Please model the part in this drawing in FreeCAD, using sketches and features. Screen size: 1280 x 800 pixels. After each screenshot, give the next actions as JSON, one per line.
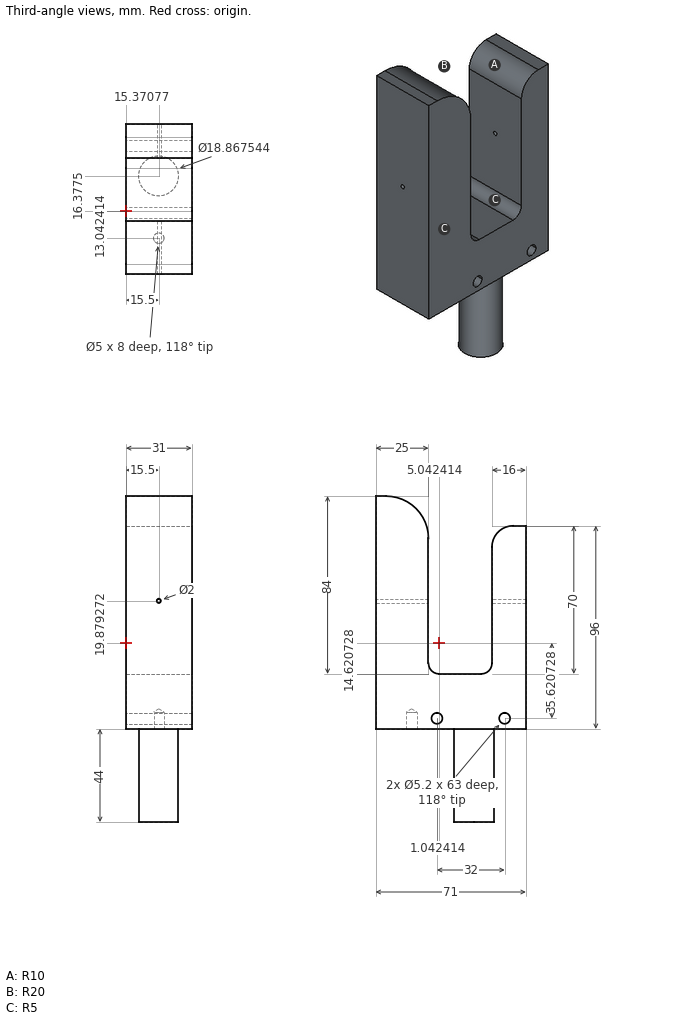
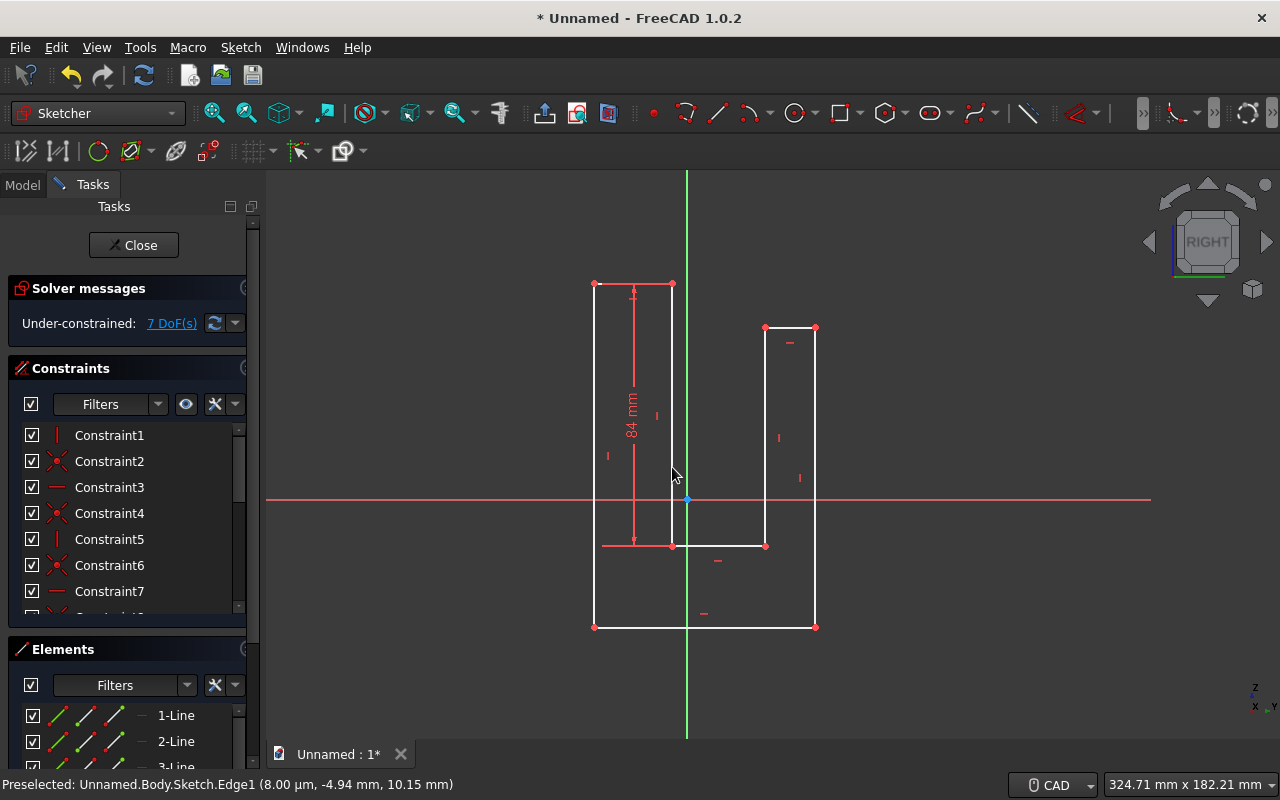
{"action": "left_click", "coordinate": [649, 284]}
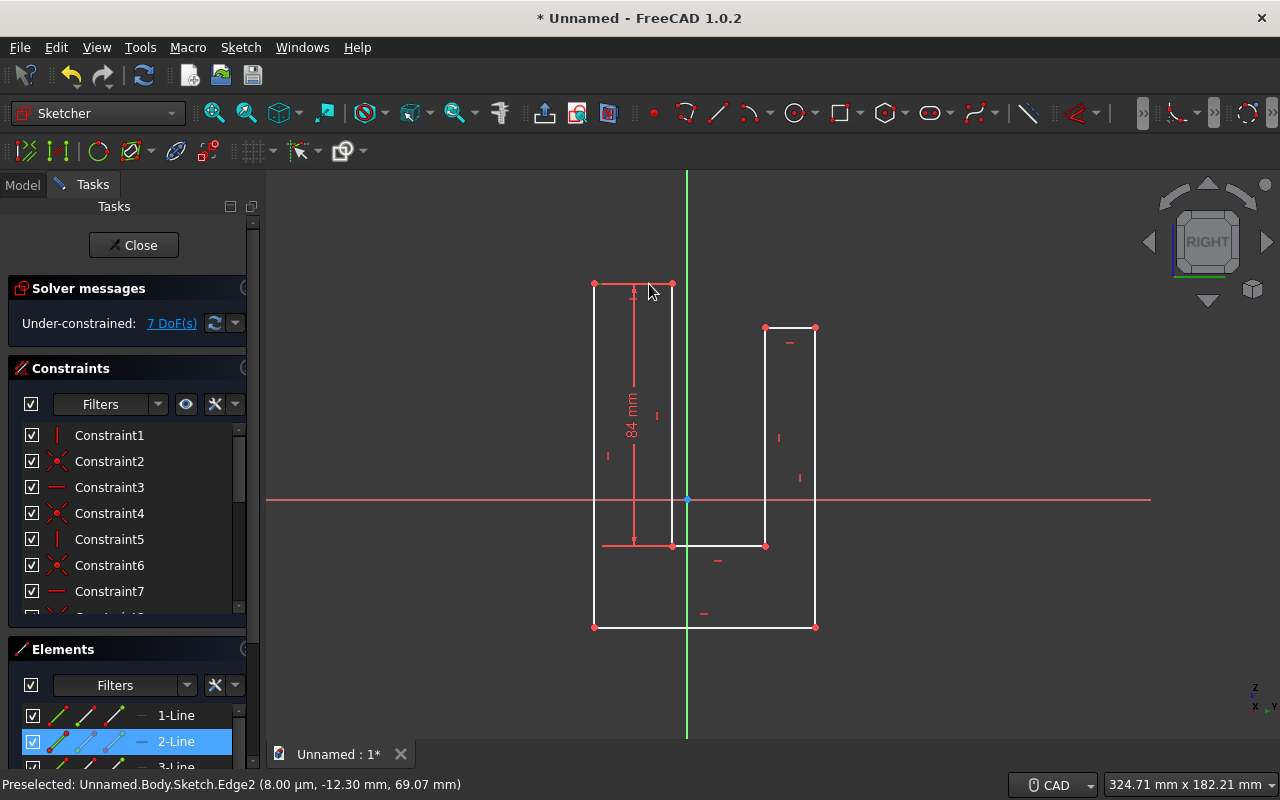
{"action": "left_click", "coordinate": [1098, 114]}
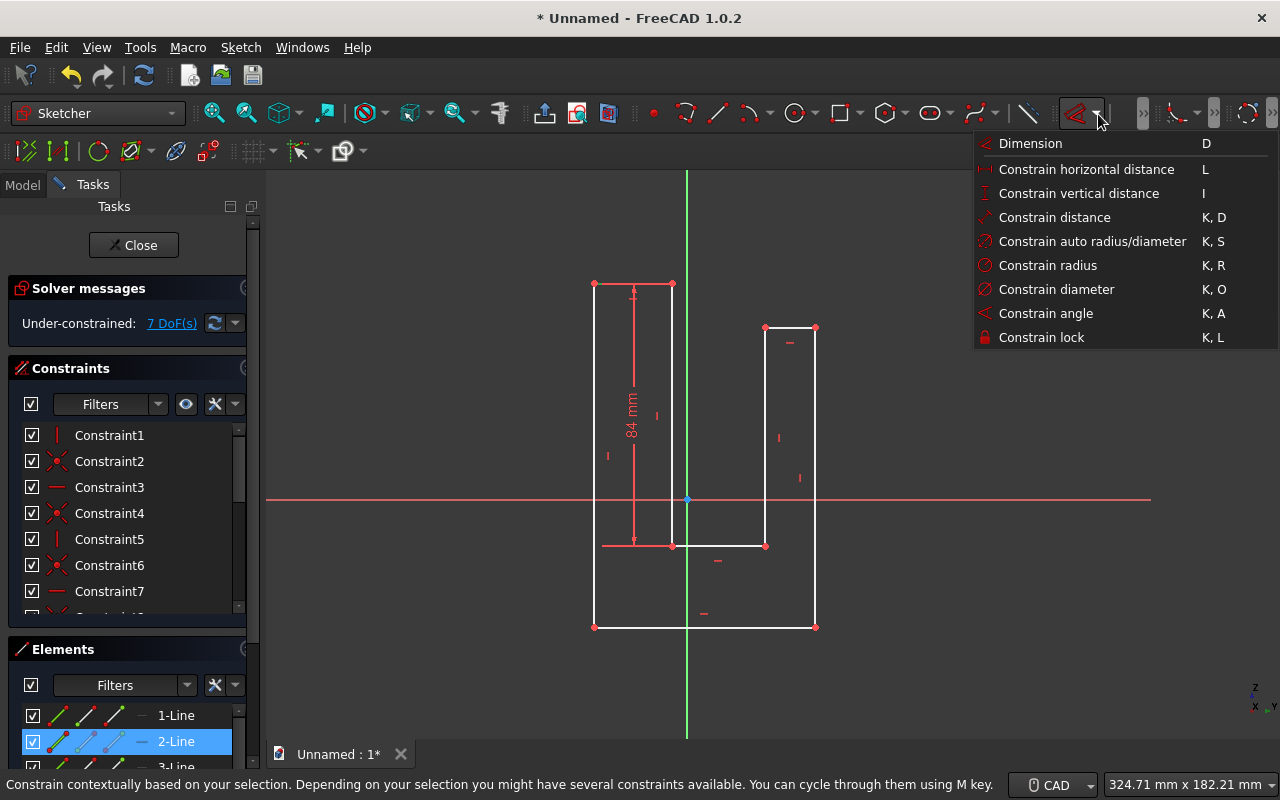
{"action": "left_click", "coordinate": [1126, 169]}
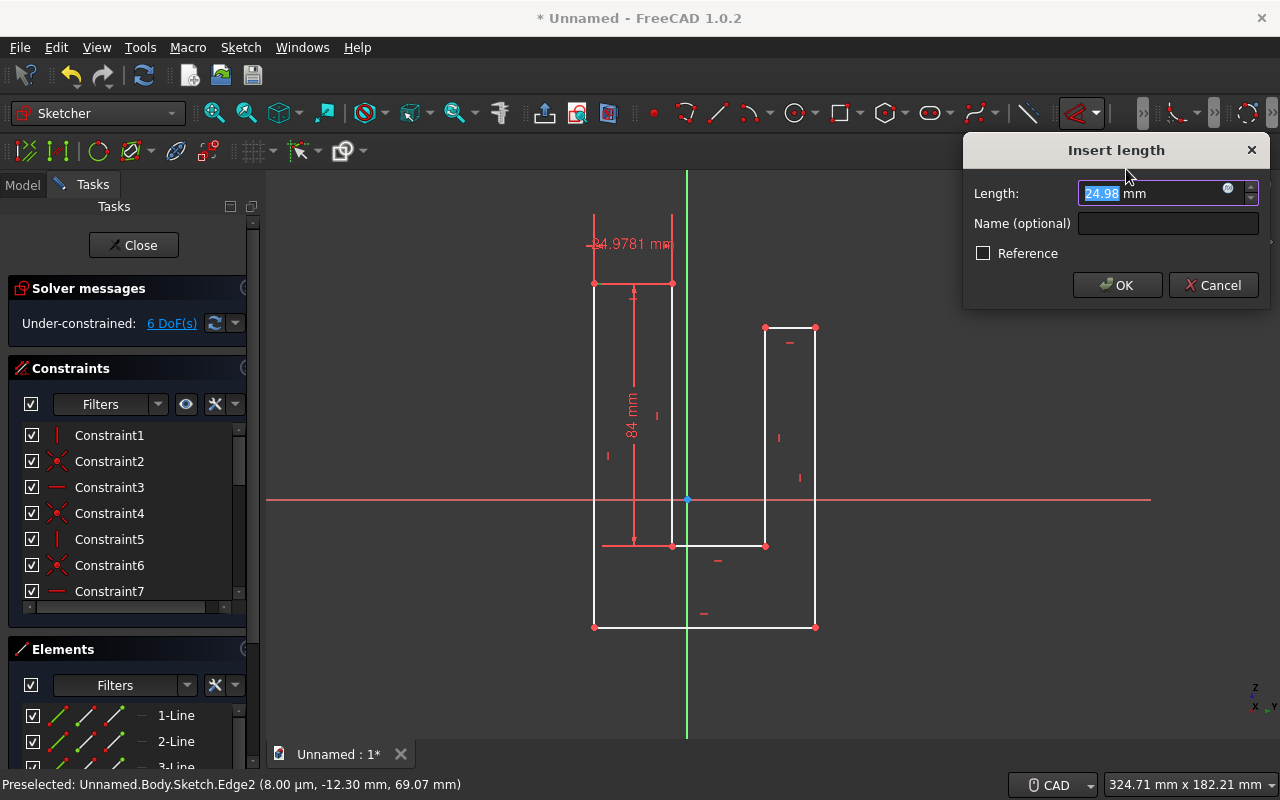
{"action": "type", "text": "25"}
{"action": "key", "text": "Return"}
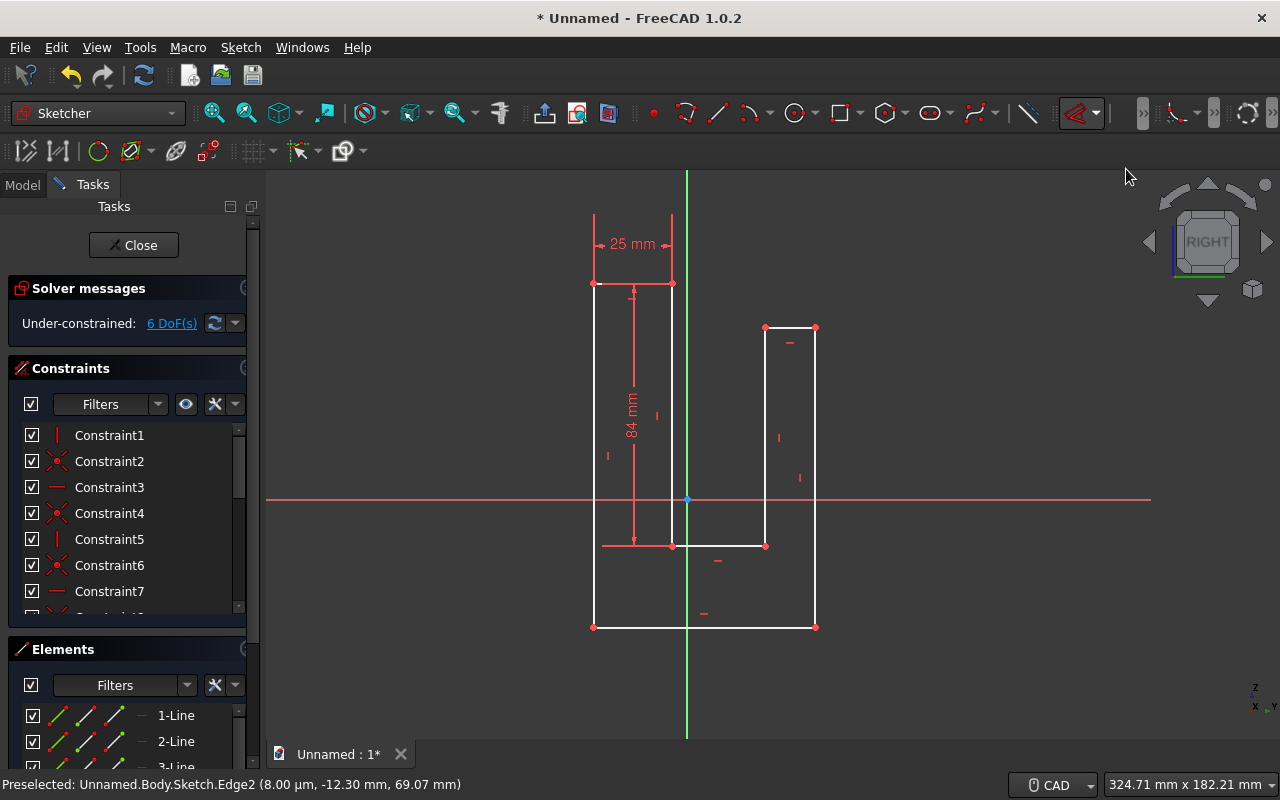
{"action": "left_click", "coordinate": [660, 628]}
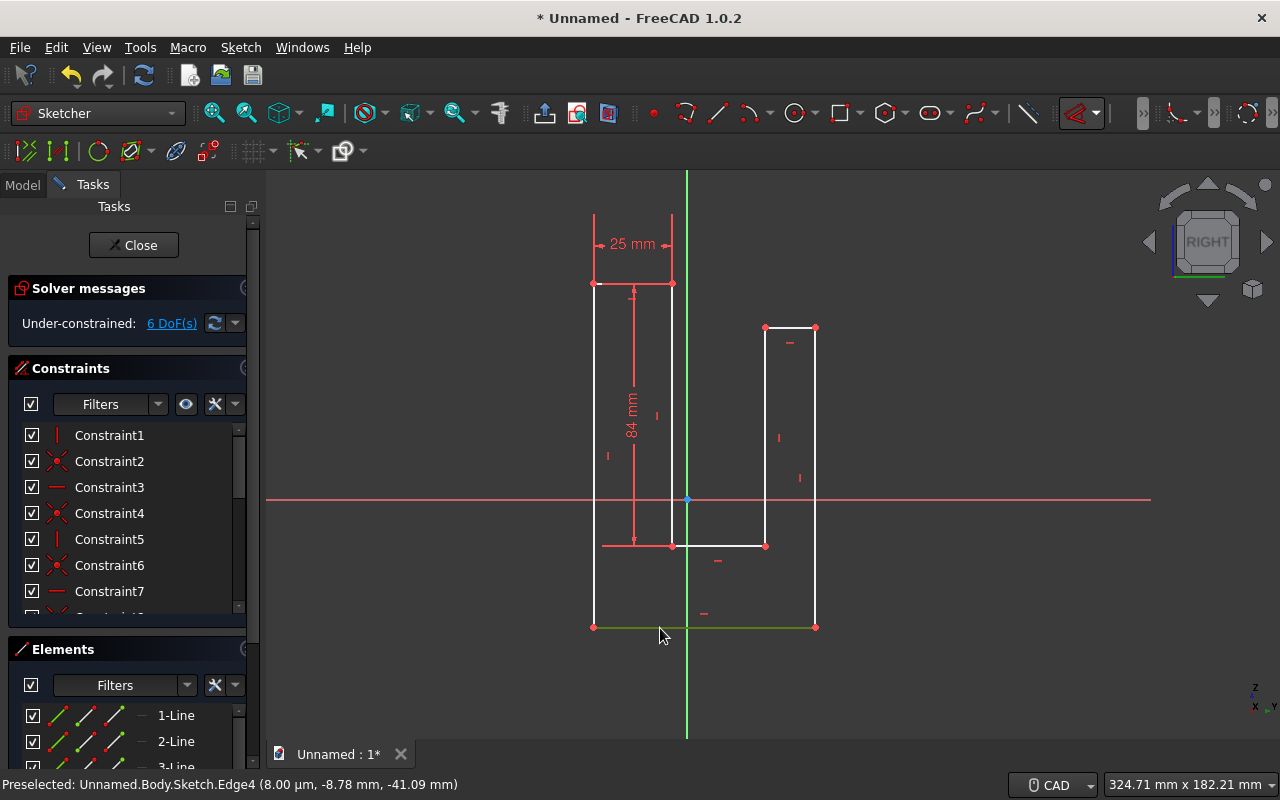
{"action": "key", "text": "l"}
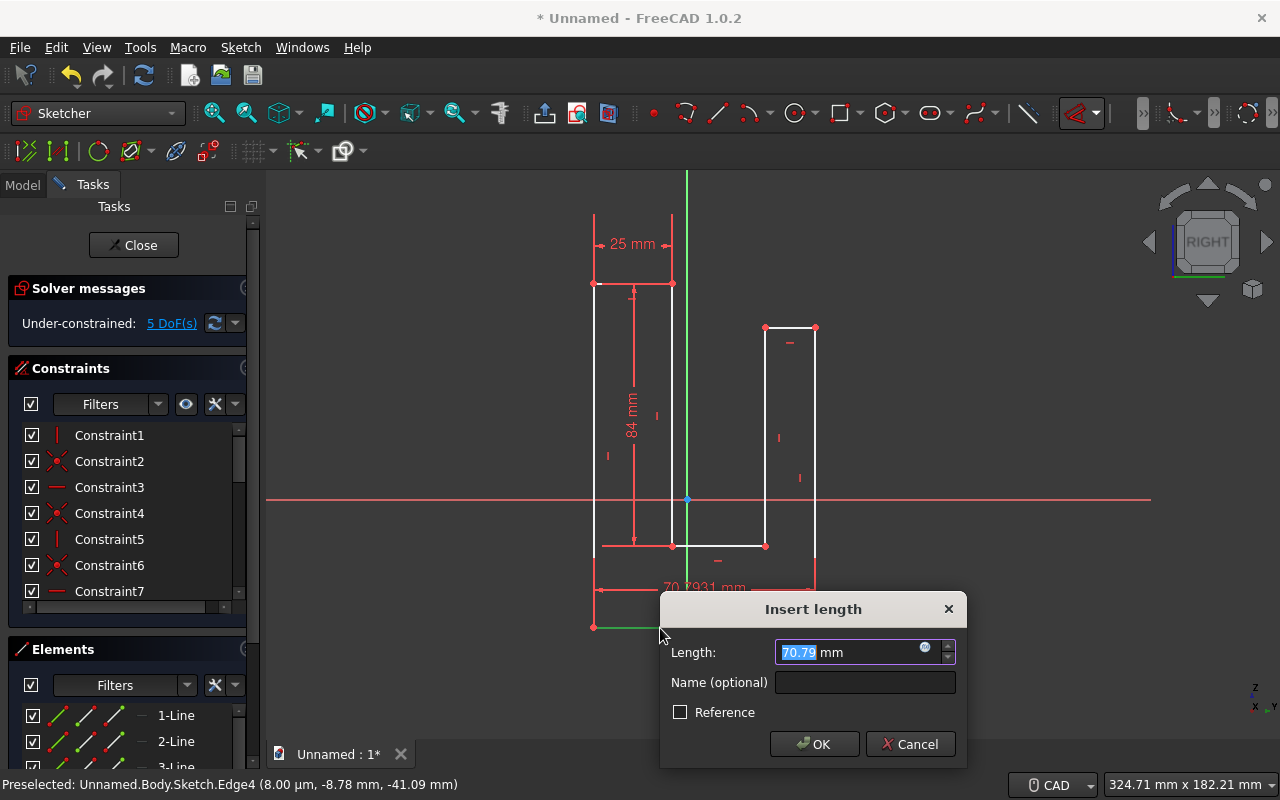
{"action": "type", "text": "71"}
{"action": "key", "text": "Return"}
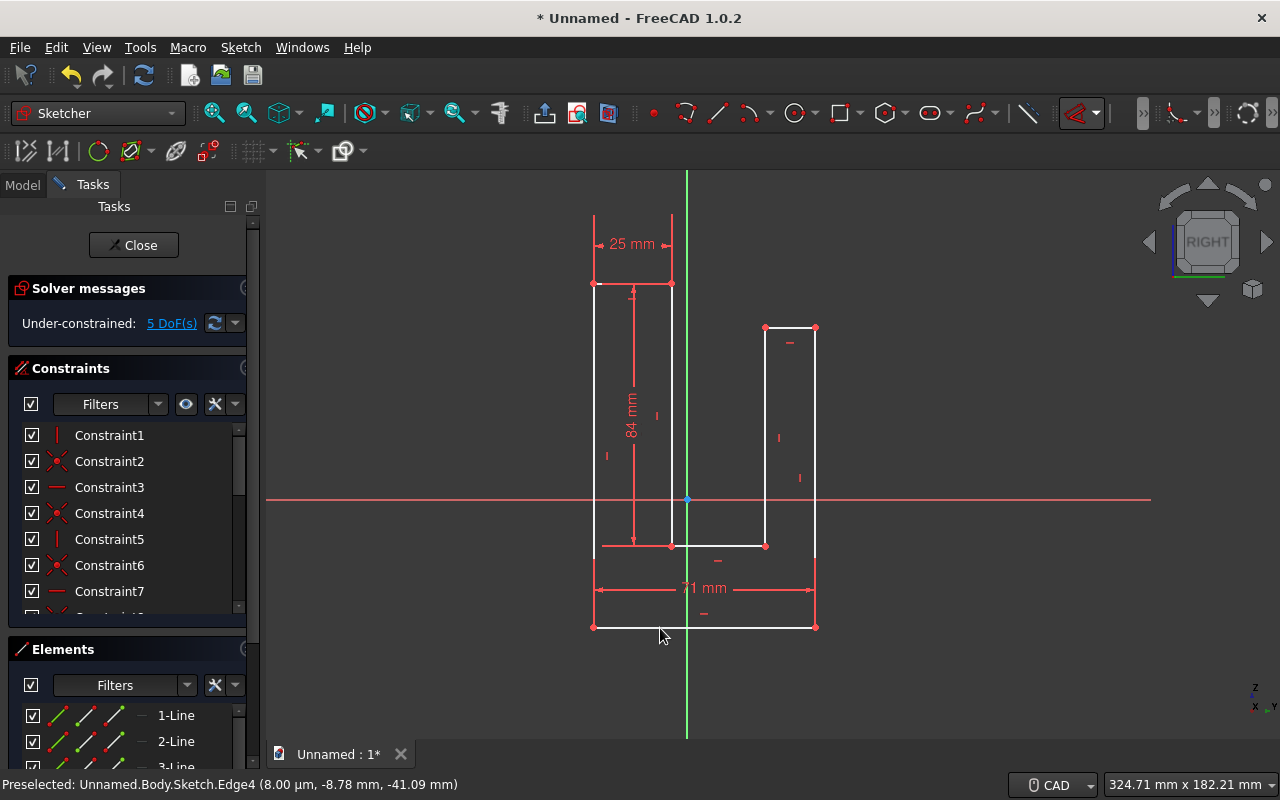
{"action": "left_click", "coordinate": [815, 538]}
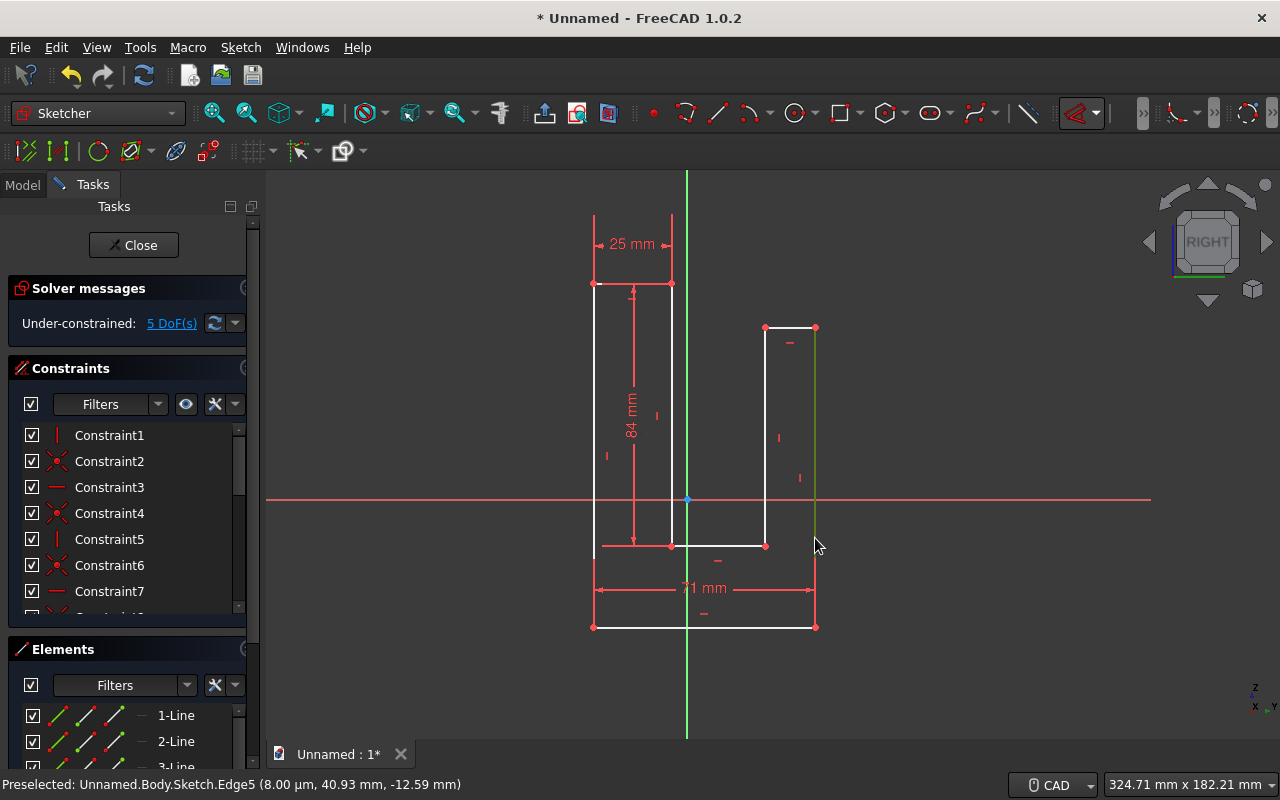
{"action": "left_click", "coordinate": [1098, 114]}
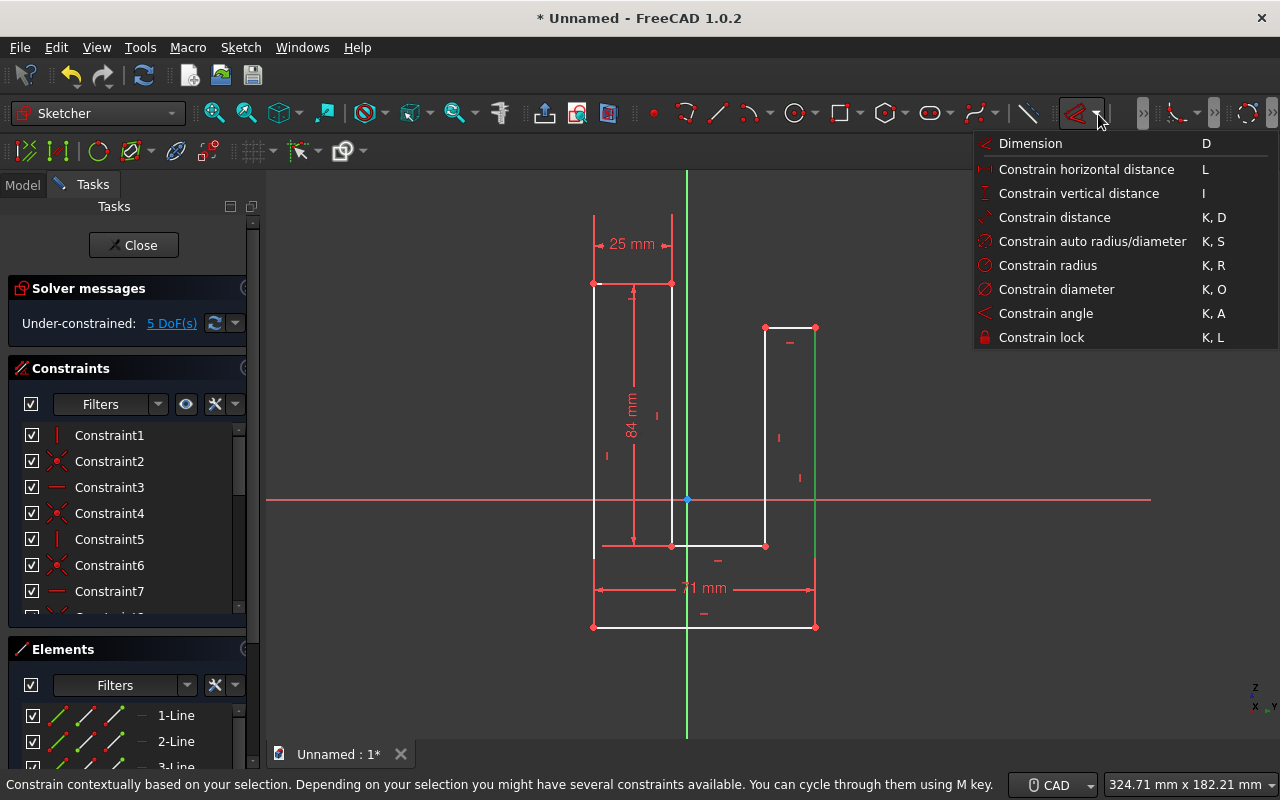
{"action": "left_click", "coordinate": [1126, 193]}